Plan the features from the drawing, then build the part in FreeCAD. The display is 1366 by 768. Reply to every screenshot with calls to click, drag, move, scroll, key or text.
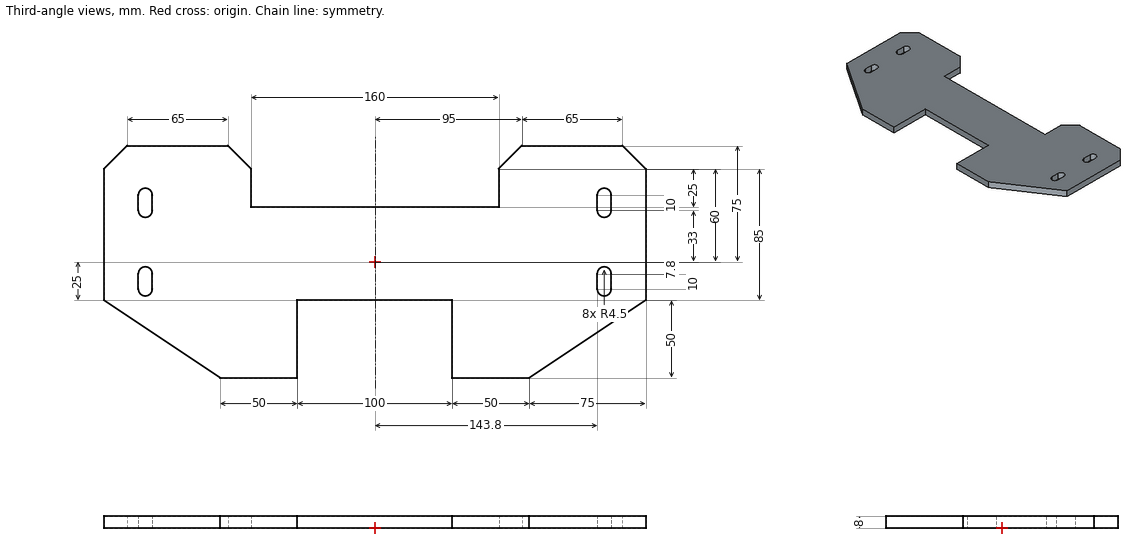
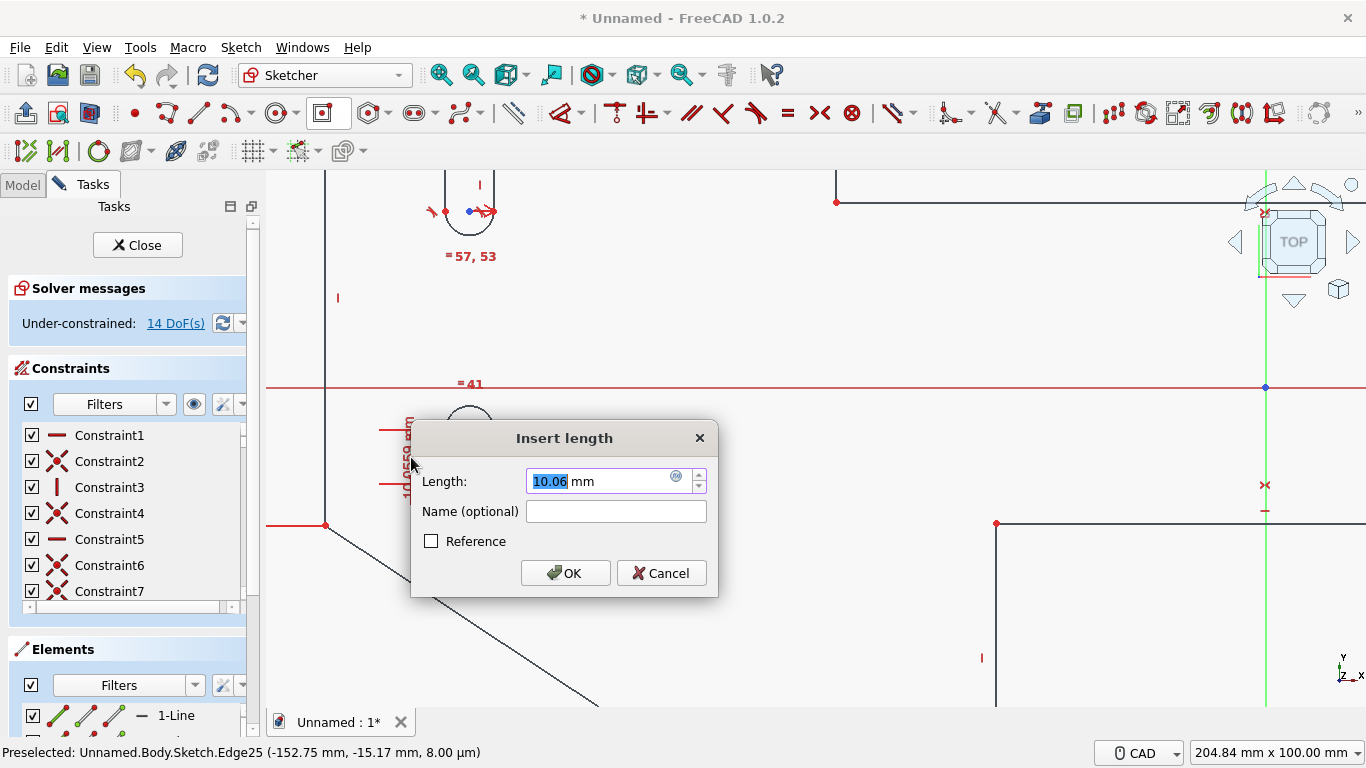
text(10)
key(Return)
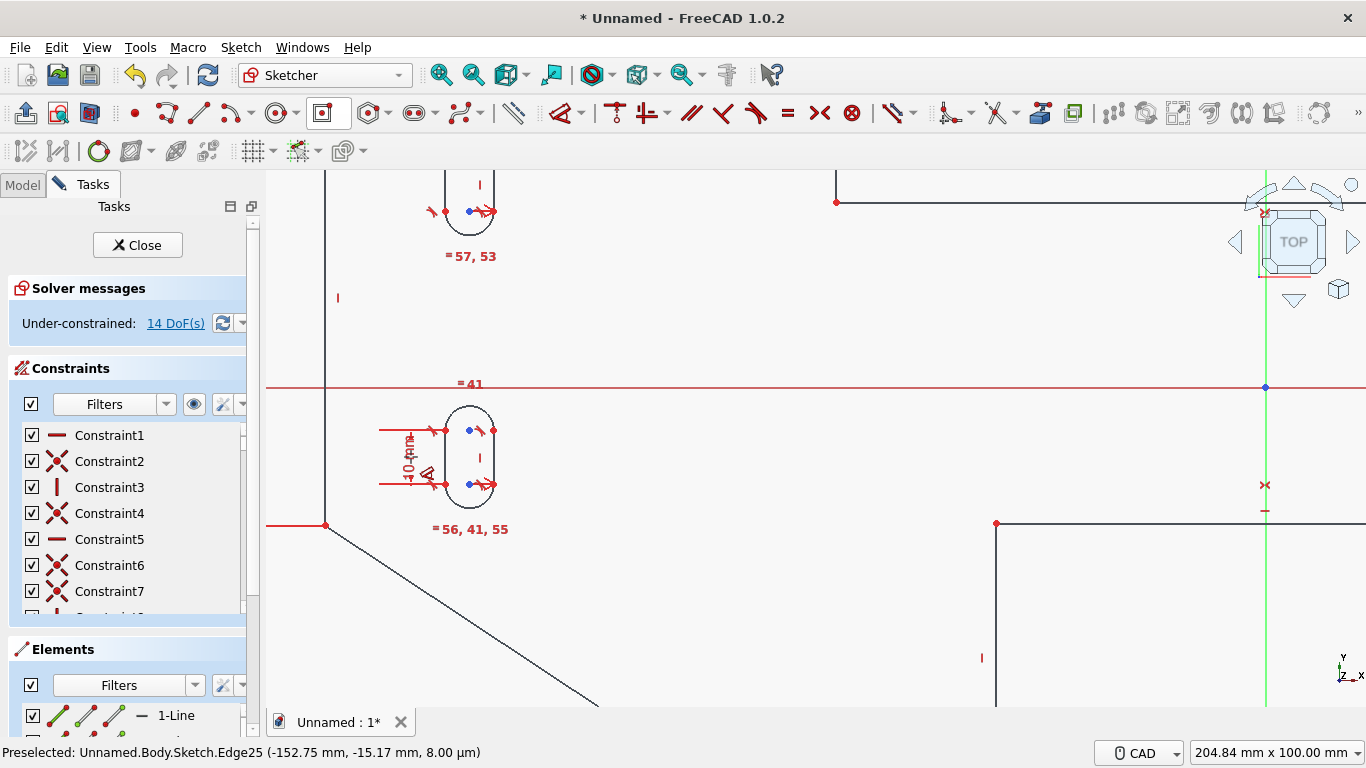
scroll(446, 468, down, 5)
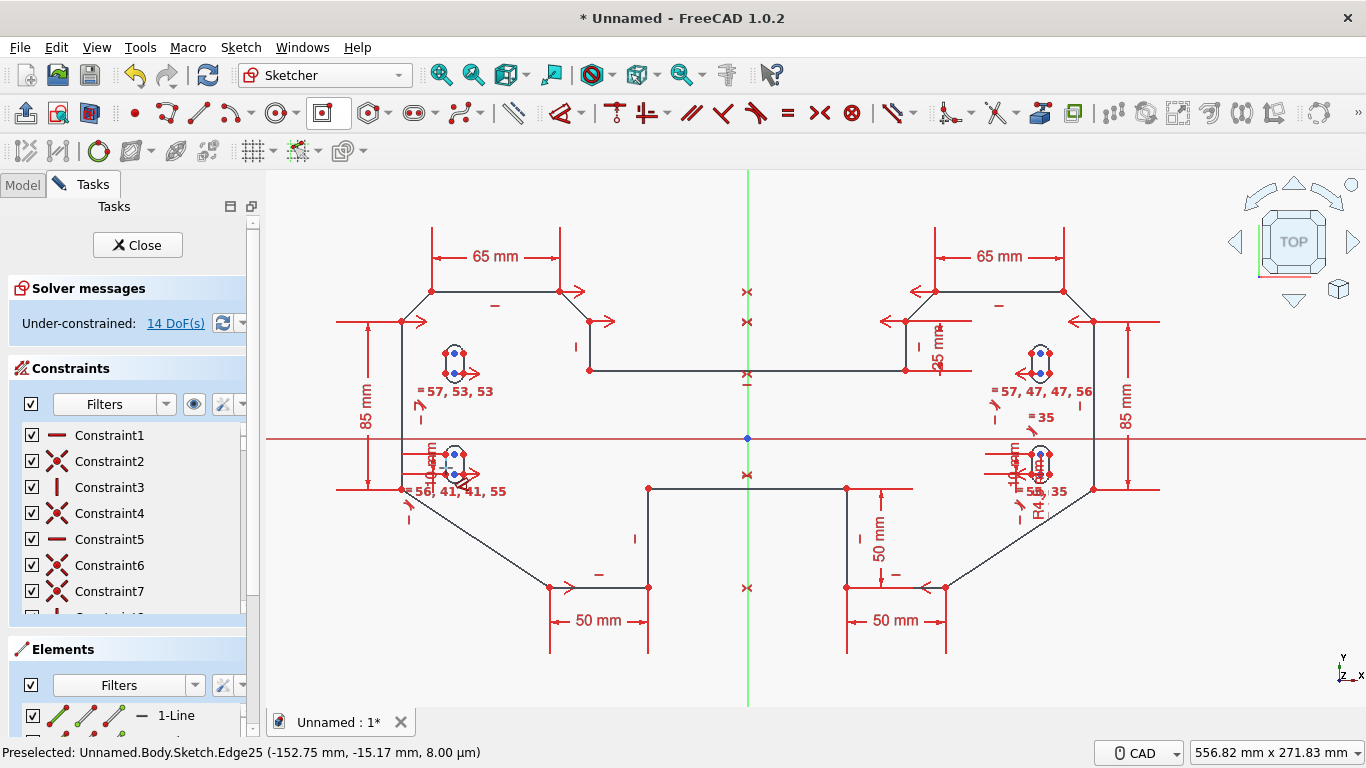
scroll(1032, 368, up, 5)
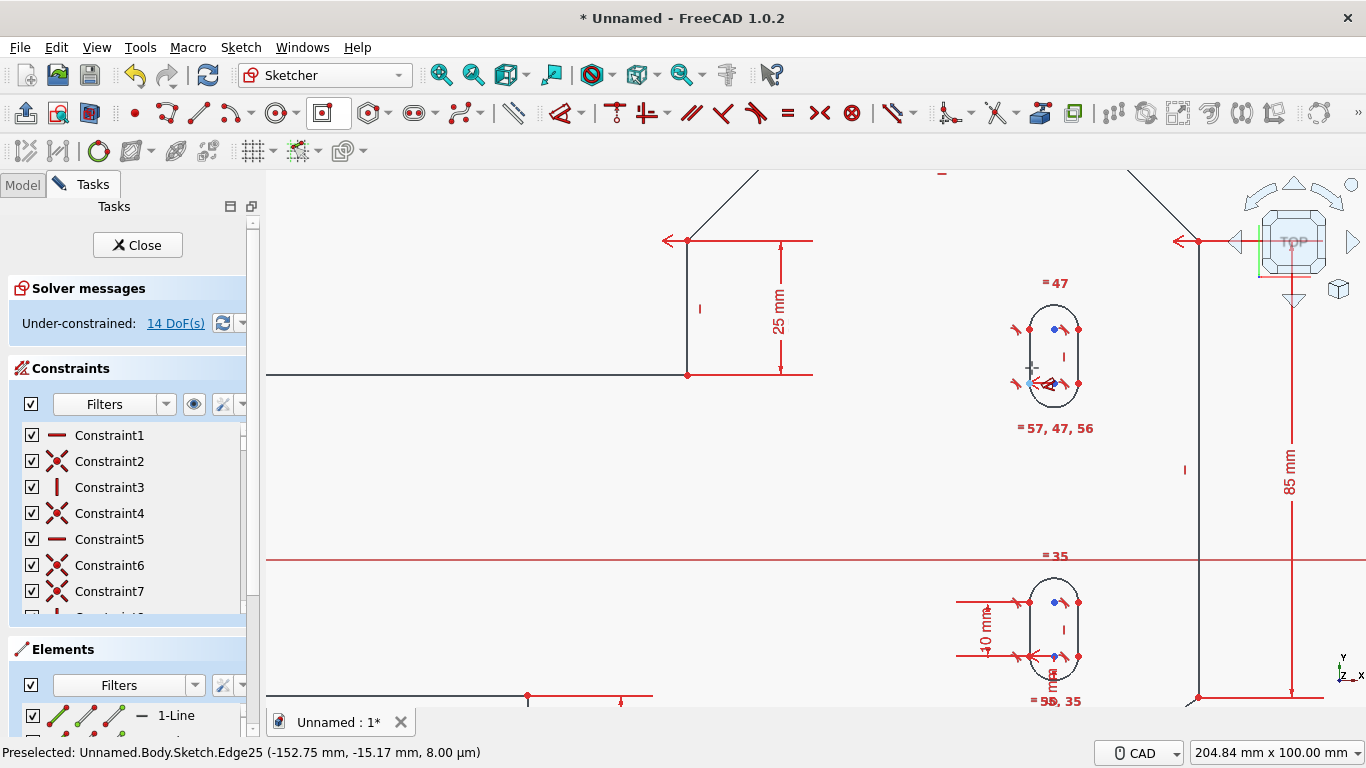
click(1030, 367)
click(1064, 356)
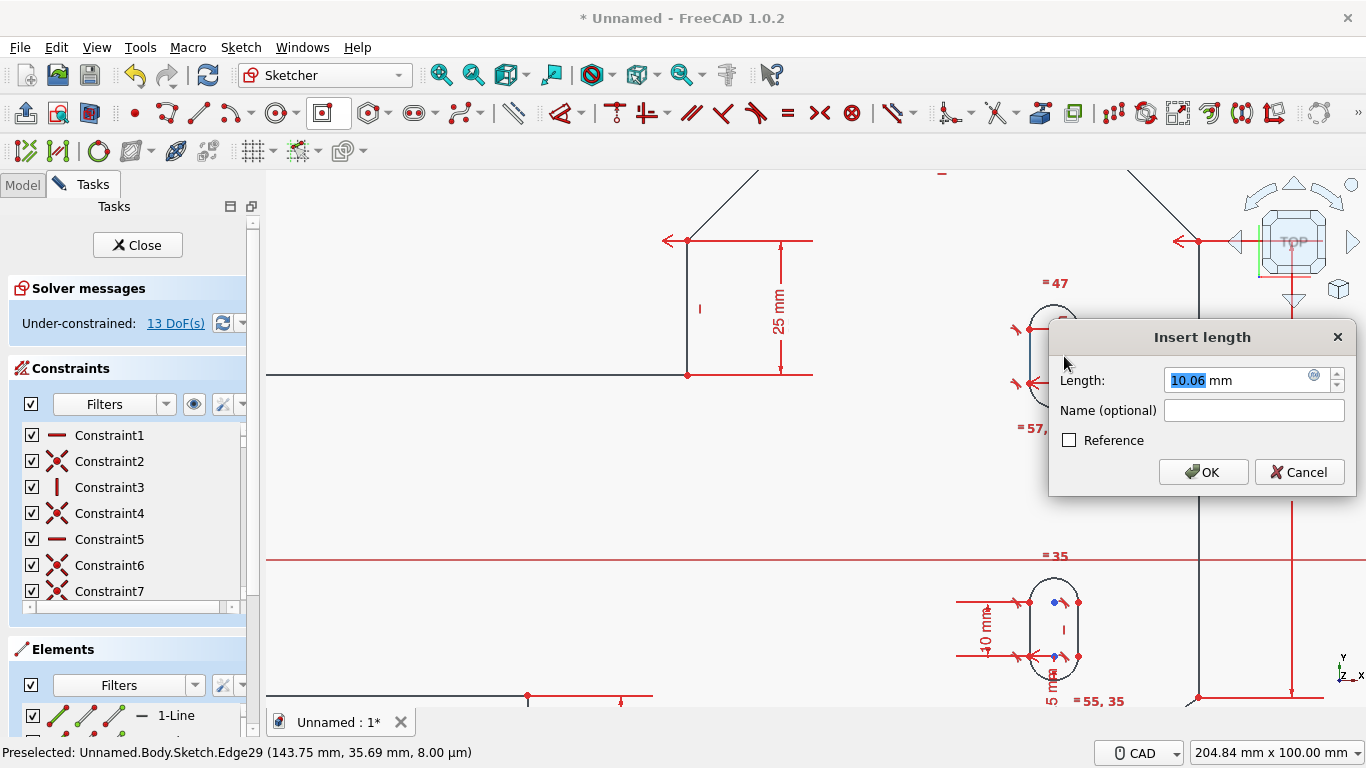
text(10)
key(Return)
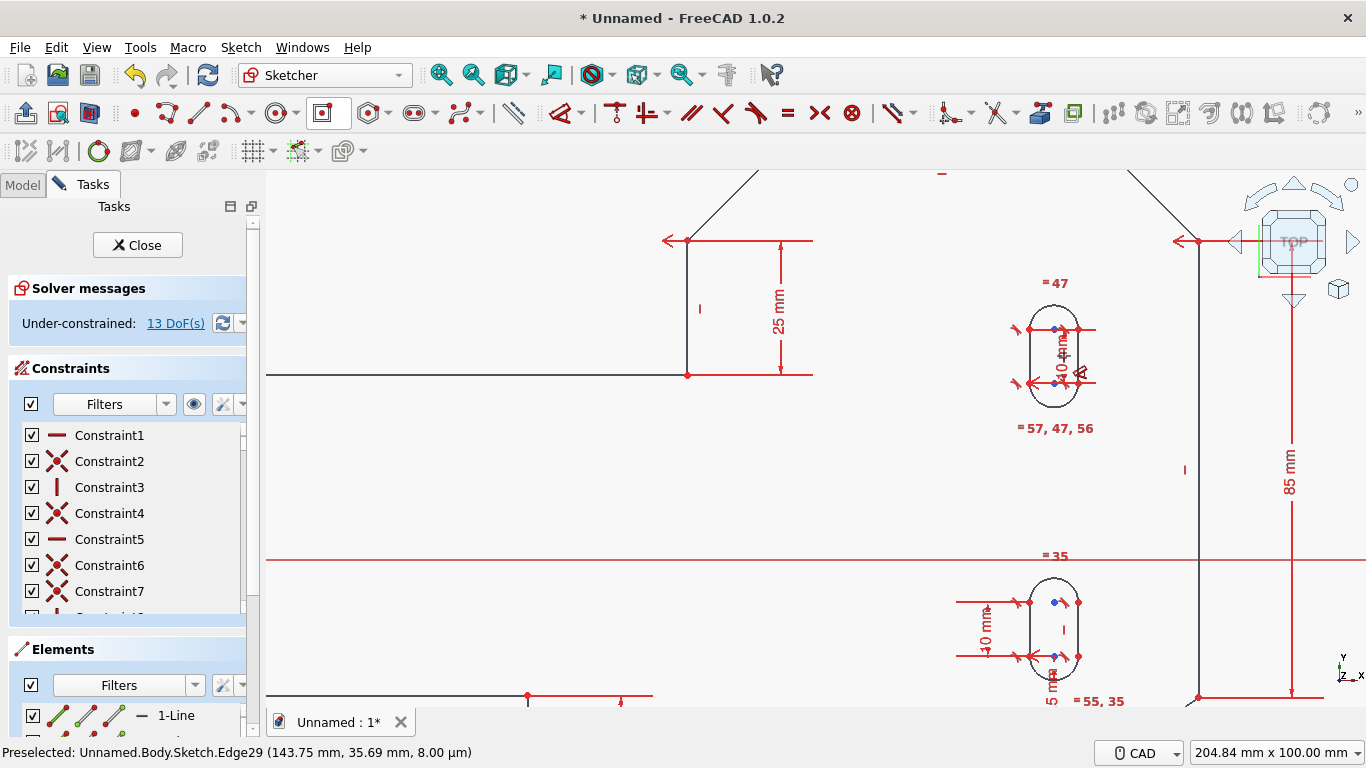
scroll(1032, 368, down, 5)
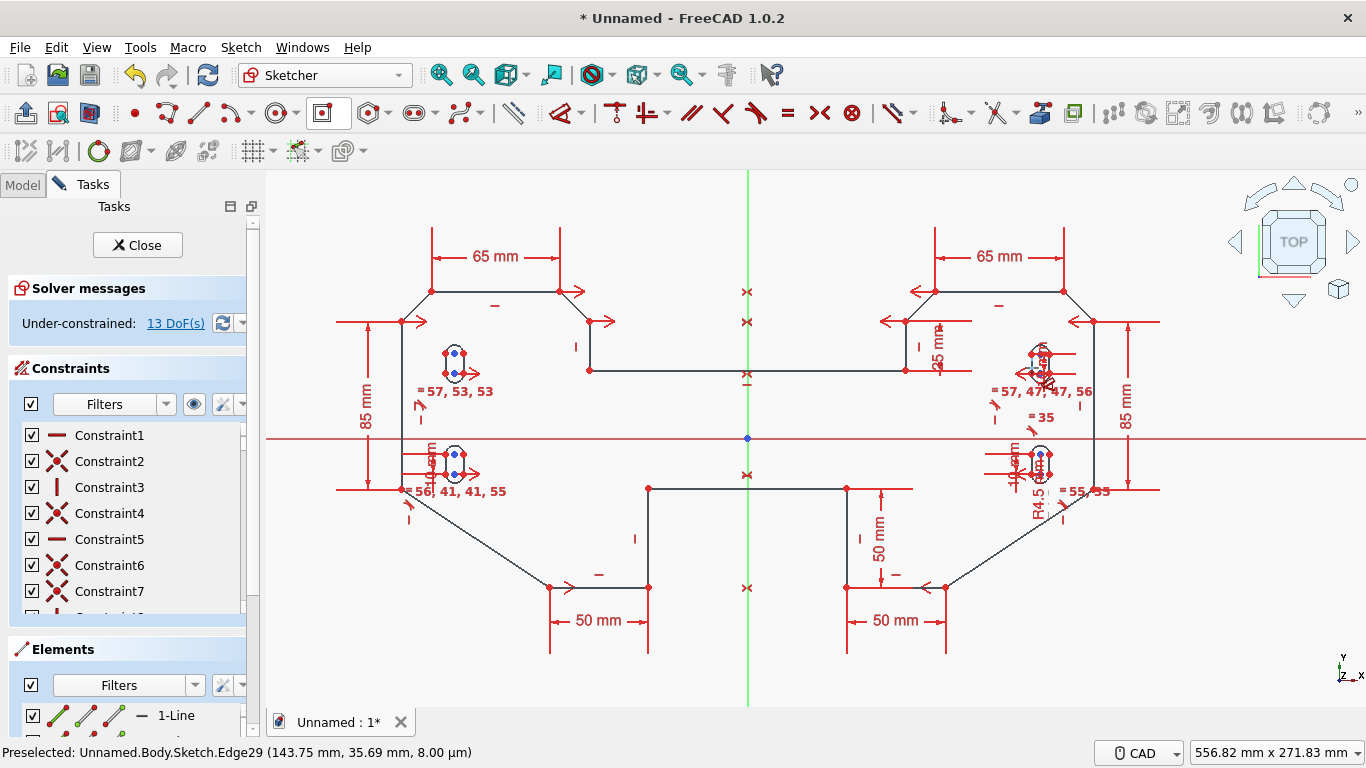
scroll(446, 368, up, 5)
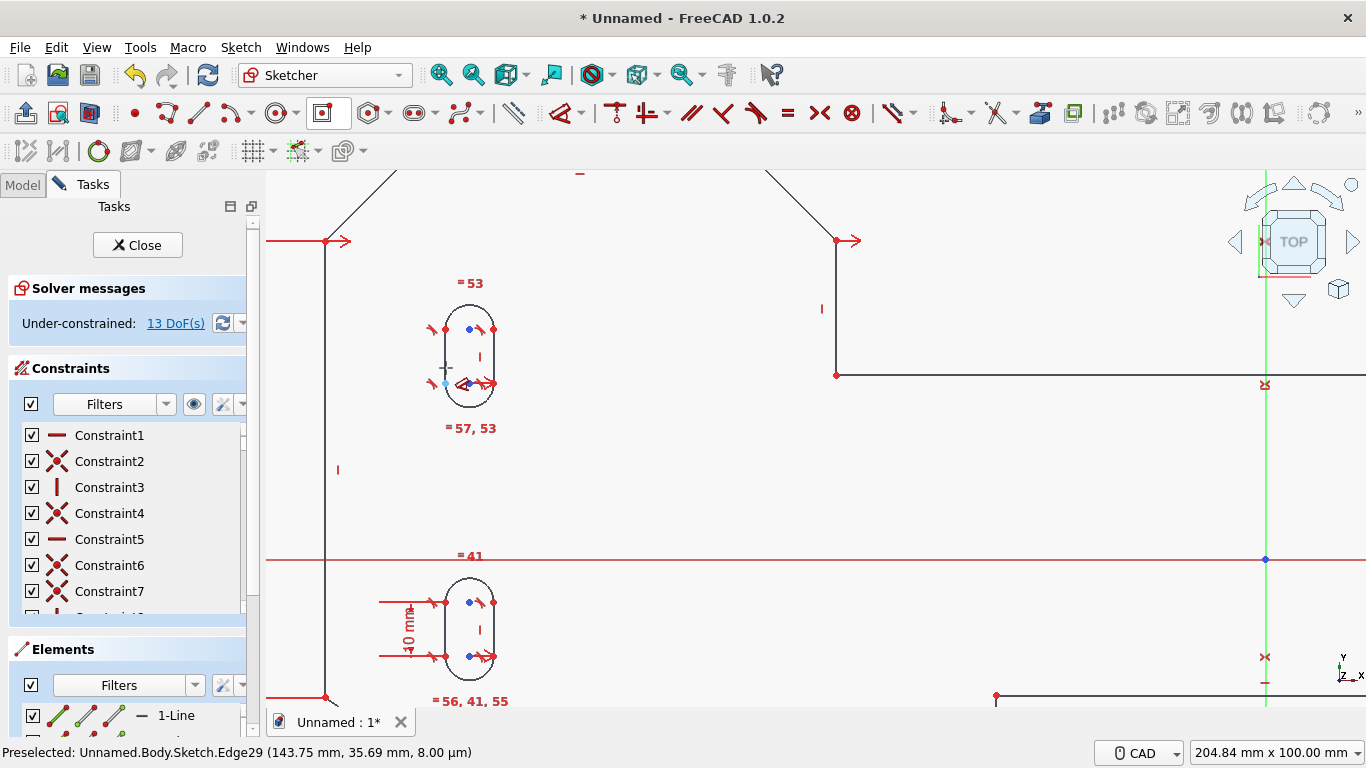
click(445, 367)
click(411, 356)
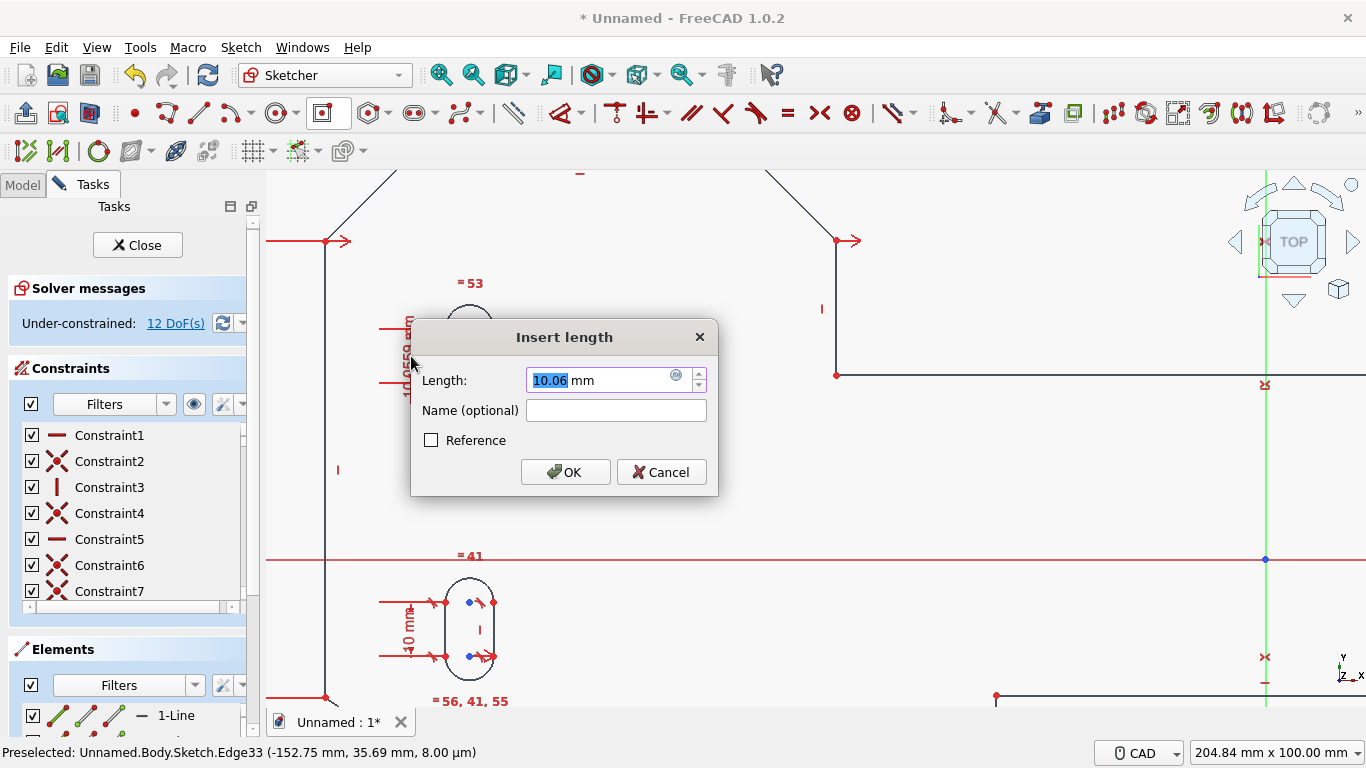
text(10)
key(Return)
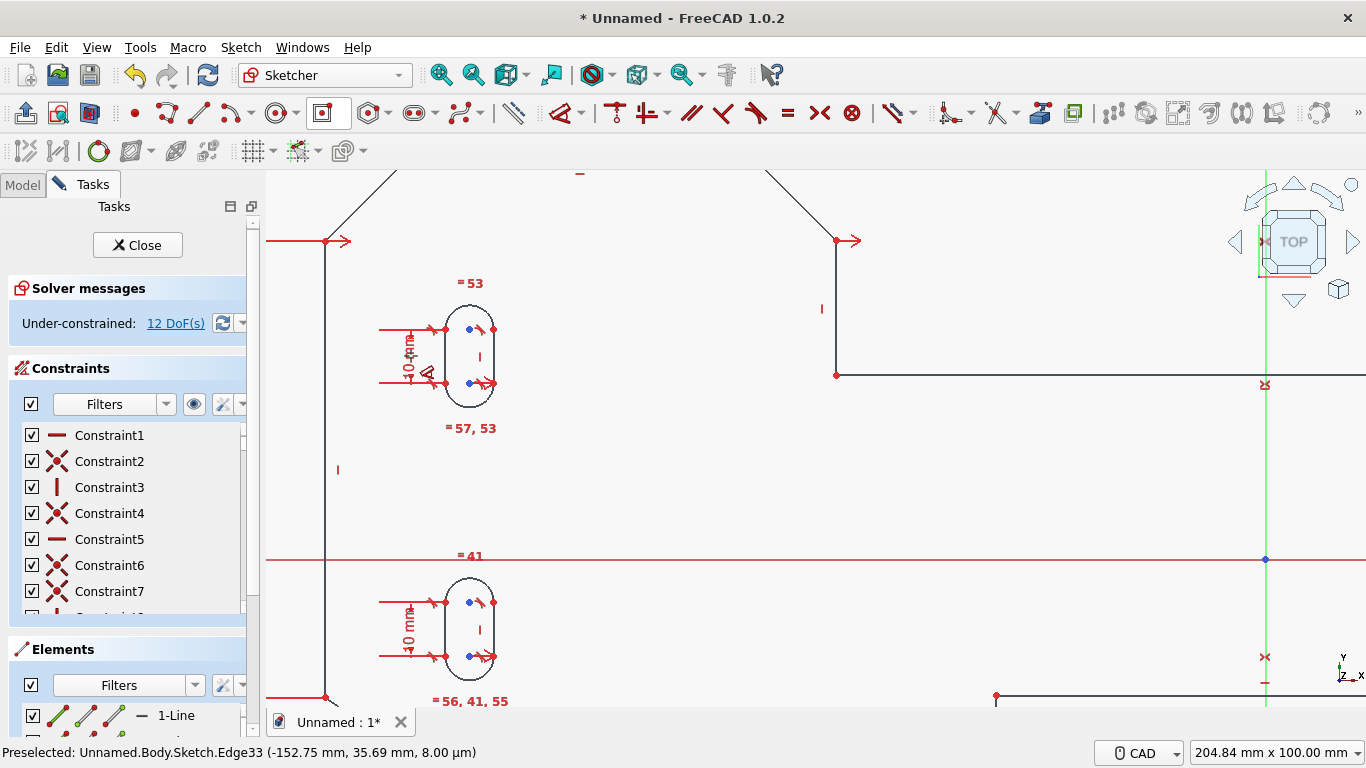
scroll(446, 368, down, 5)